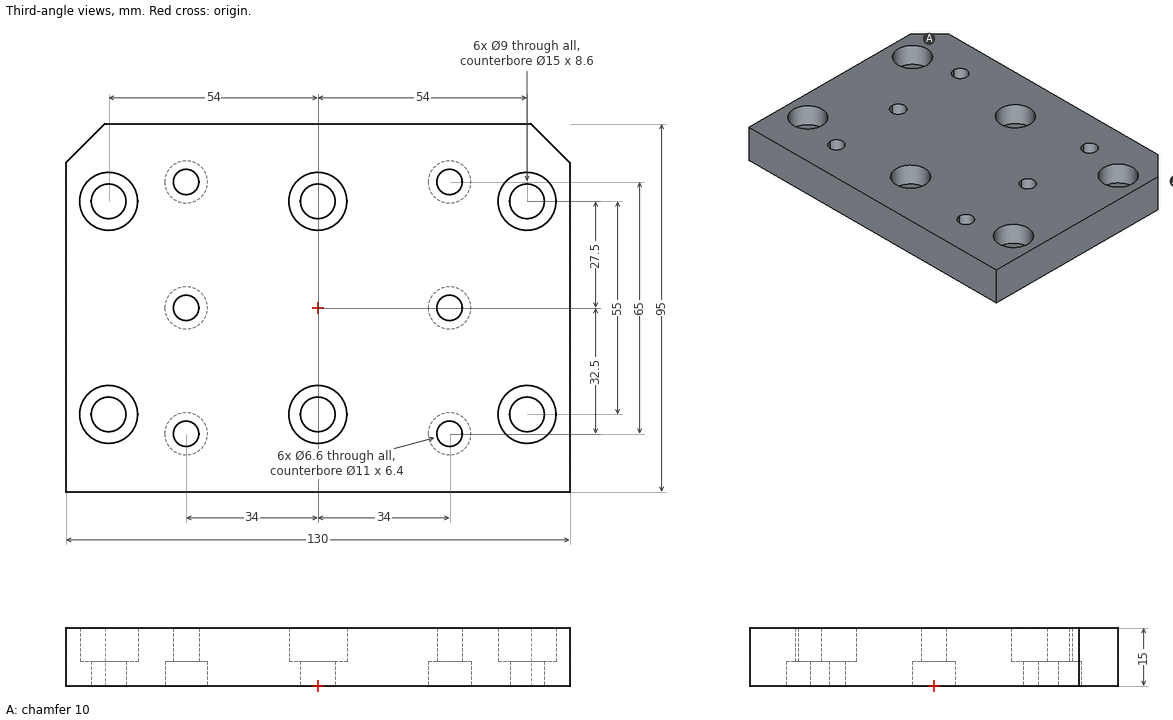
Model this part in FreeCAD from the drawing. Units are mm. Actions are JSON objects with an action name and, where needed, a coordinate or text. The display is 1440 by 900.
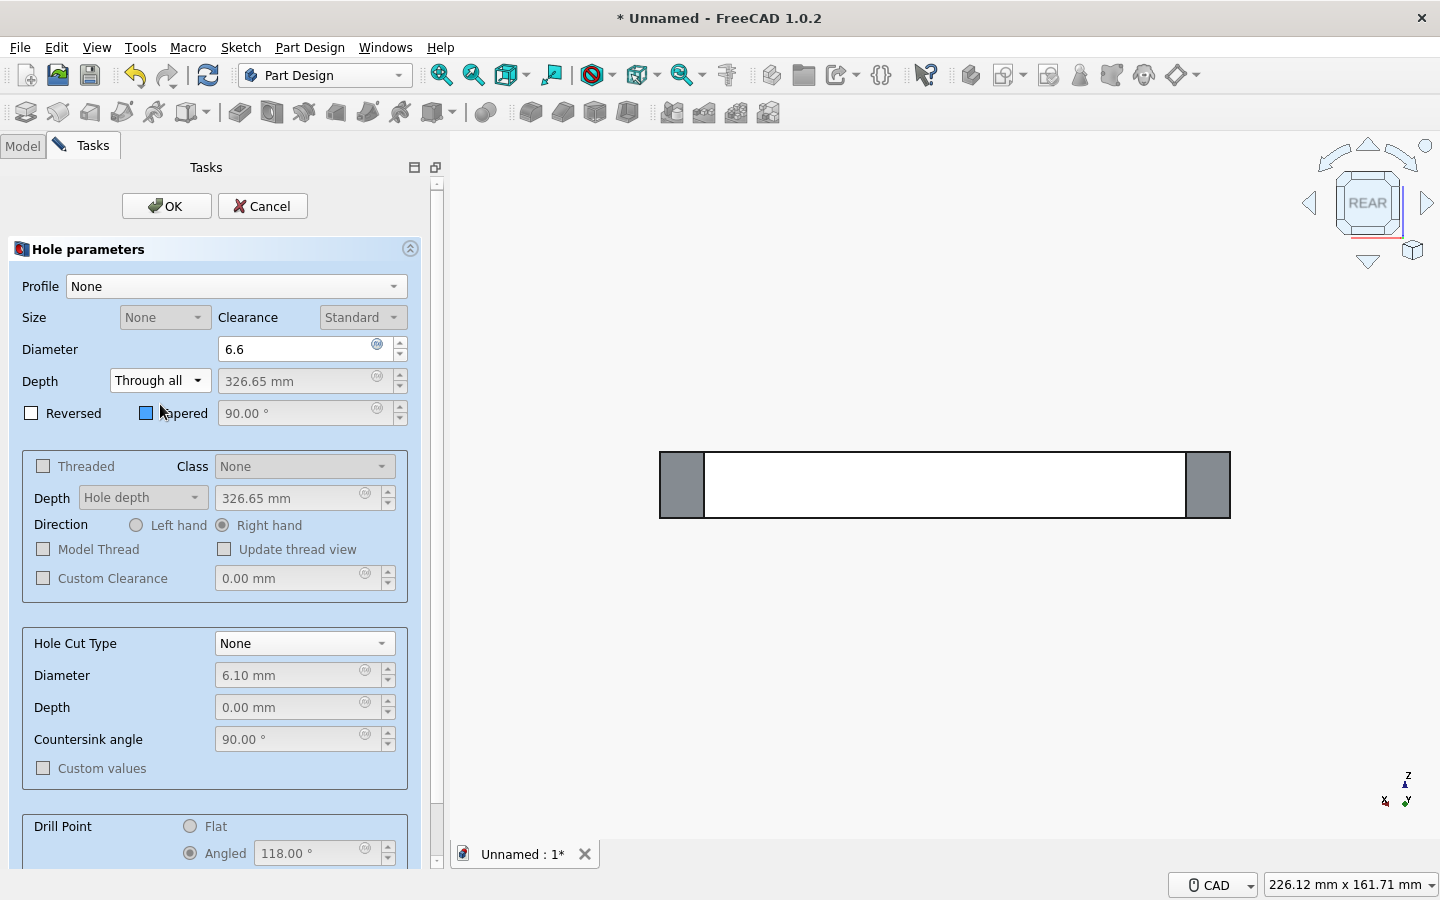
{"action": "left_click", "coordinate": [30, 413]}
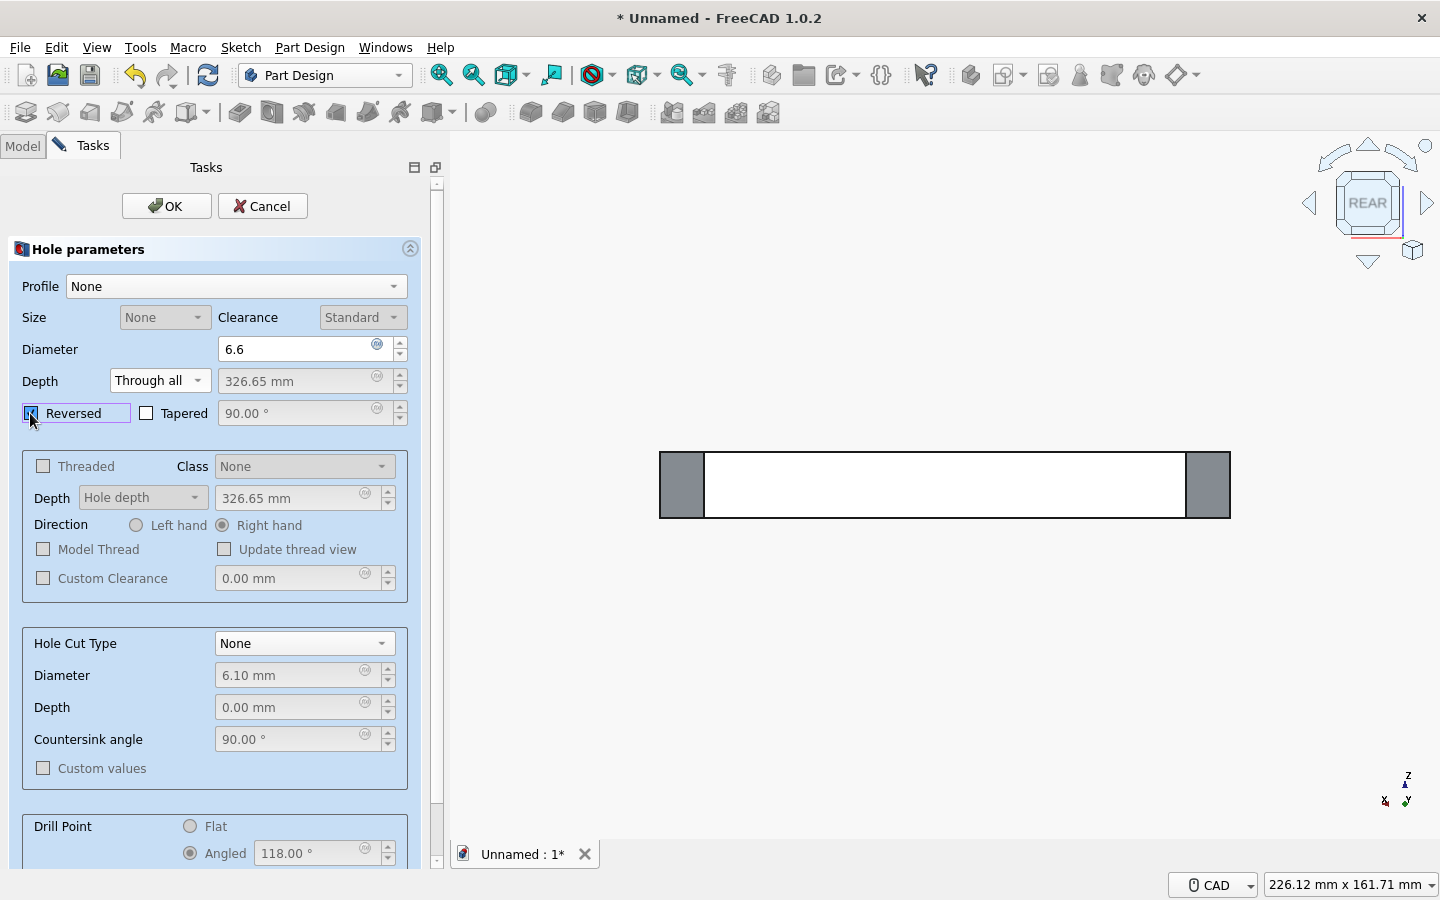
{"action": "left_click", "coordinate": [306, 644]}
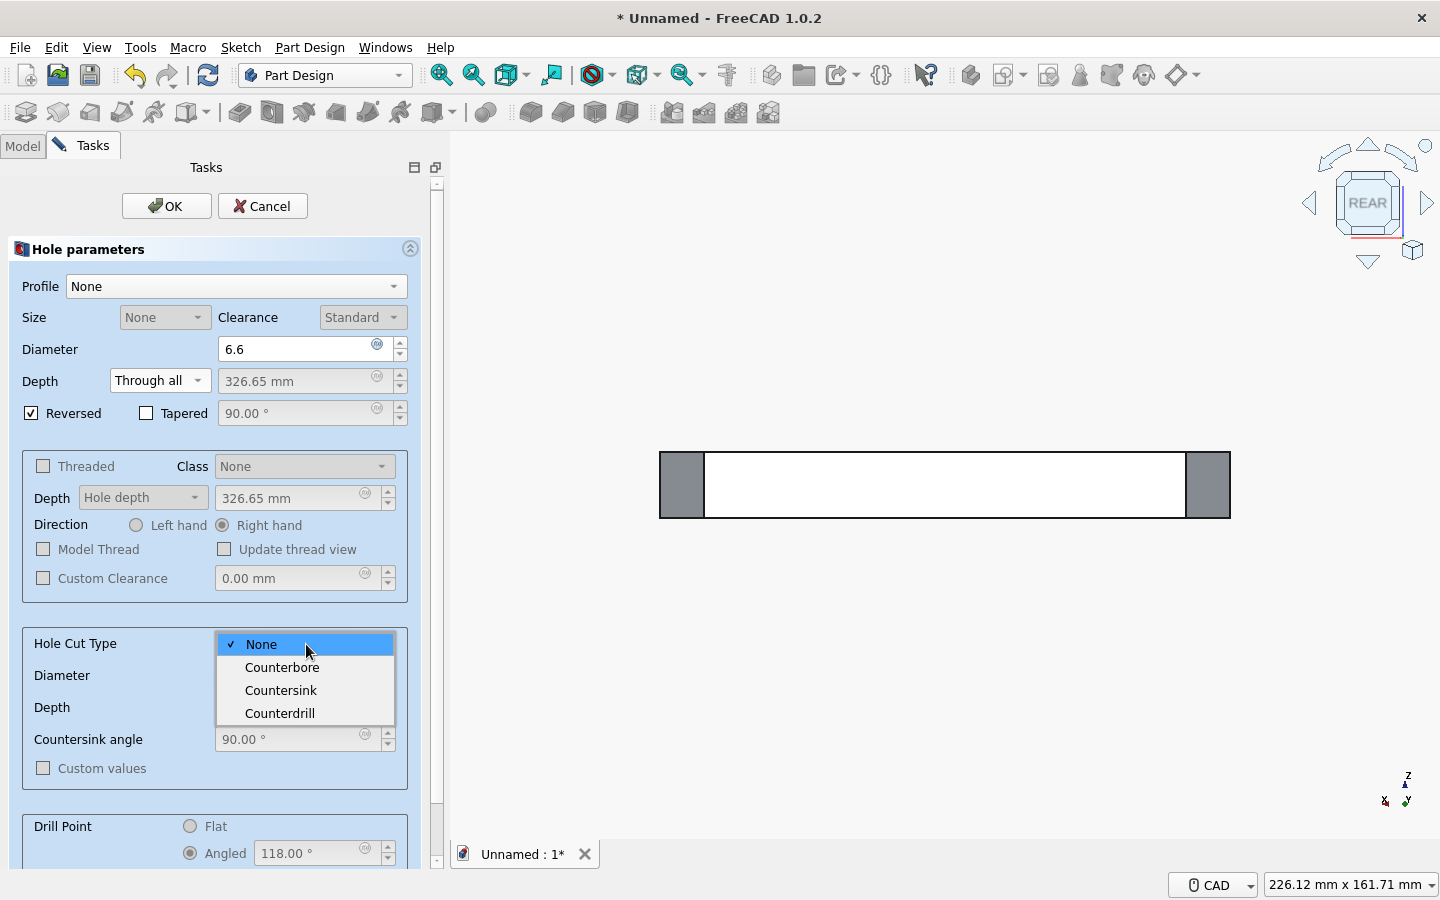
{"action": "left_click", "coordinate": [304, 668]}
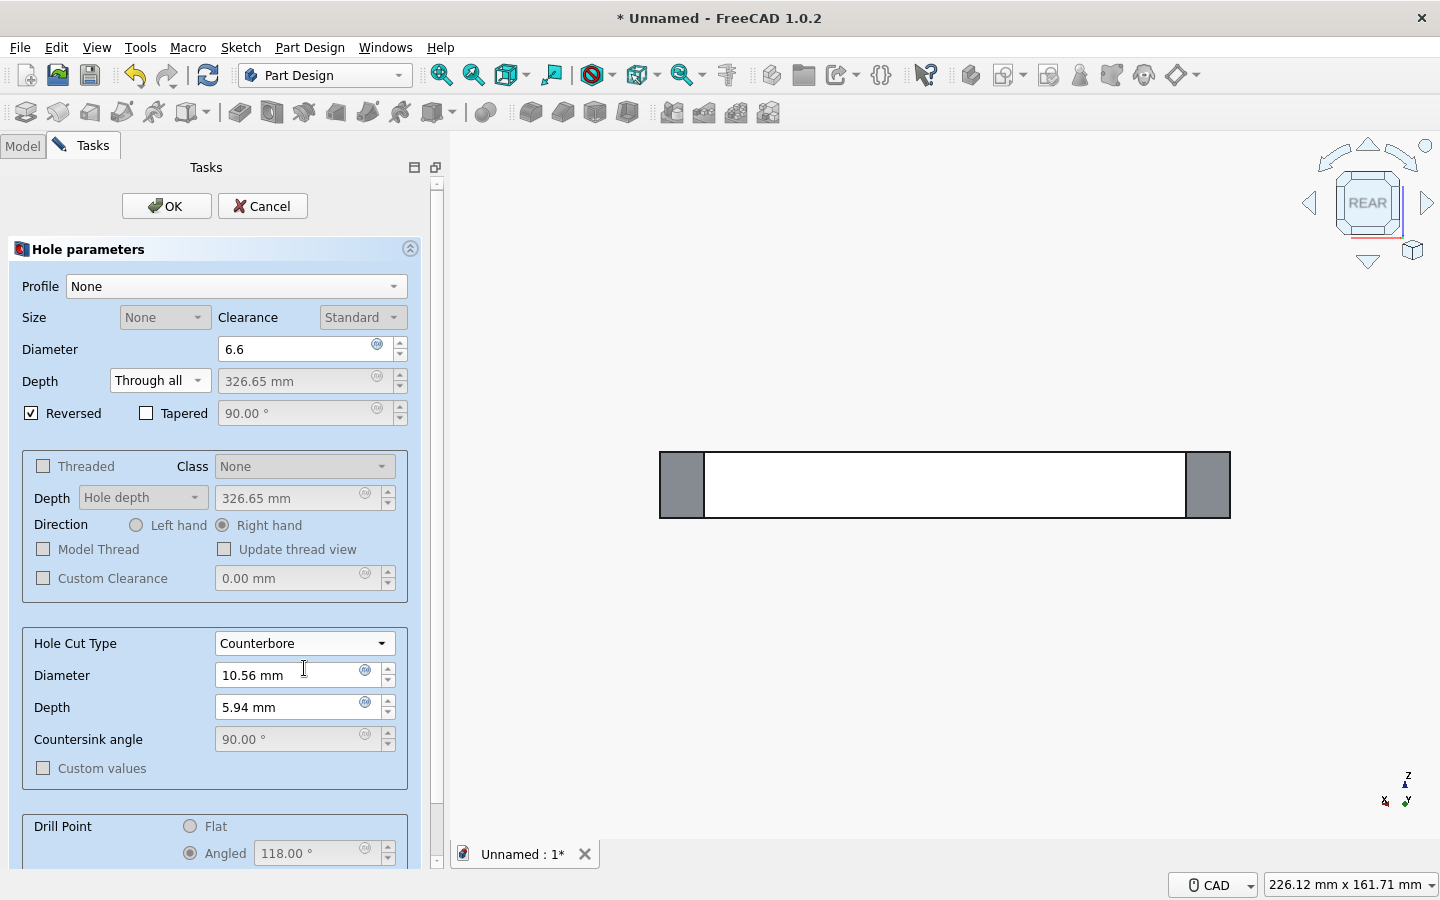
{"action": "triple_click", "coordinate": [298, 675]}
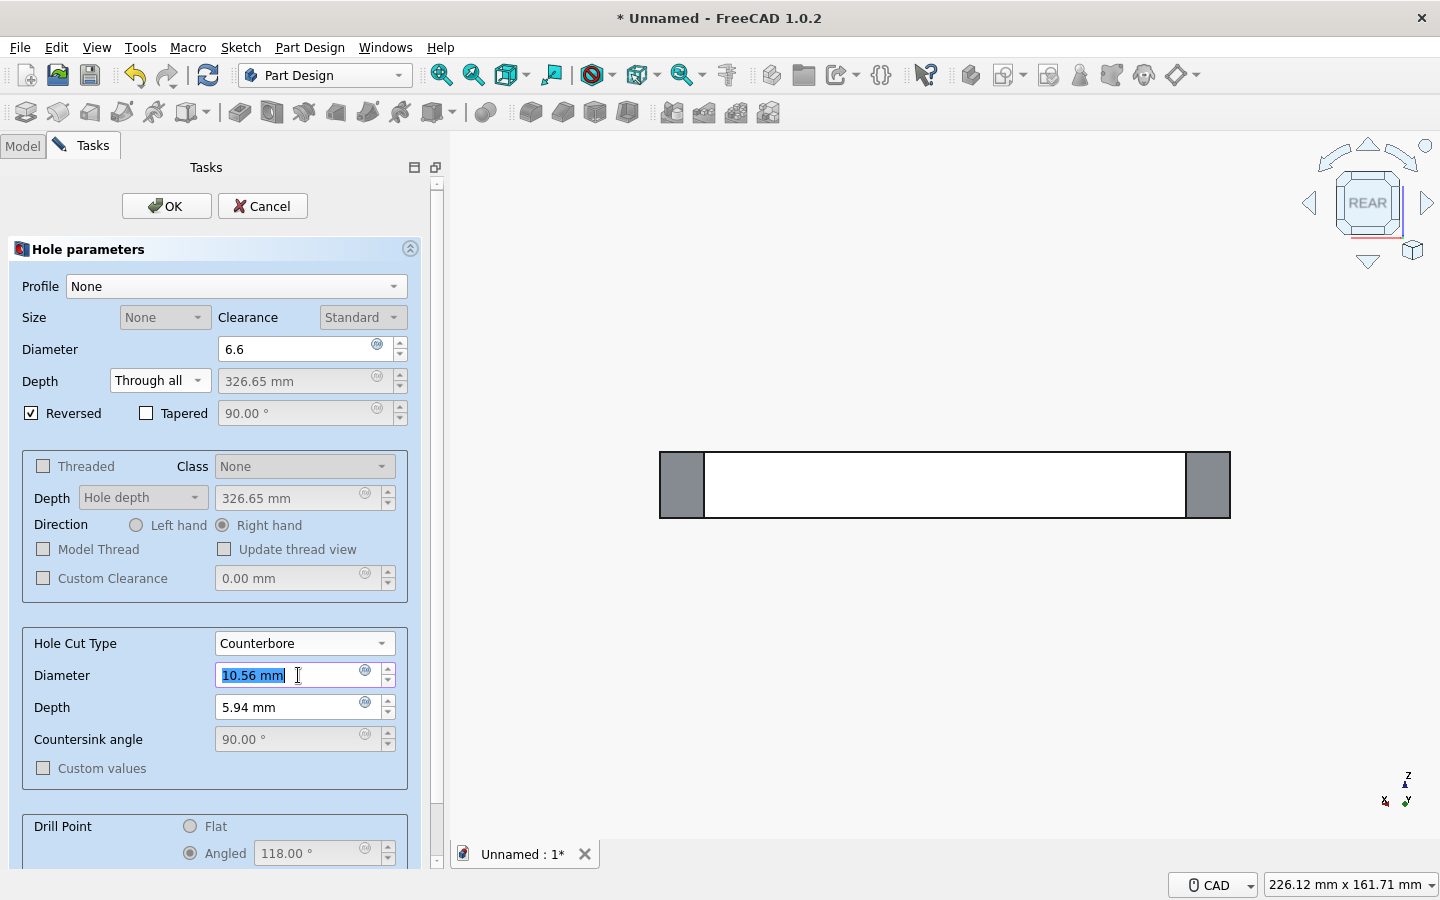
{"action": "type", "text": "11"}
{"action": "key", "text": "Tab"}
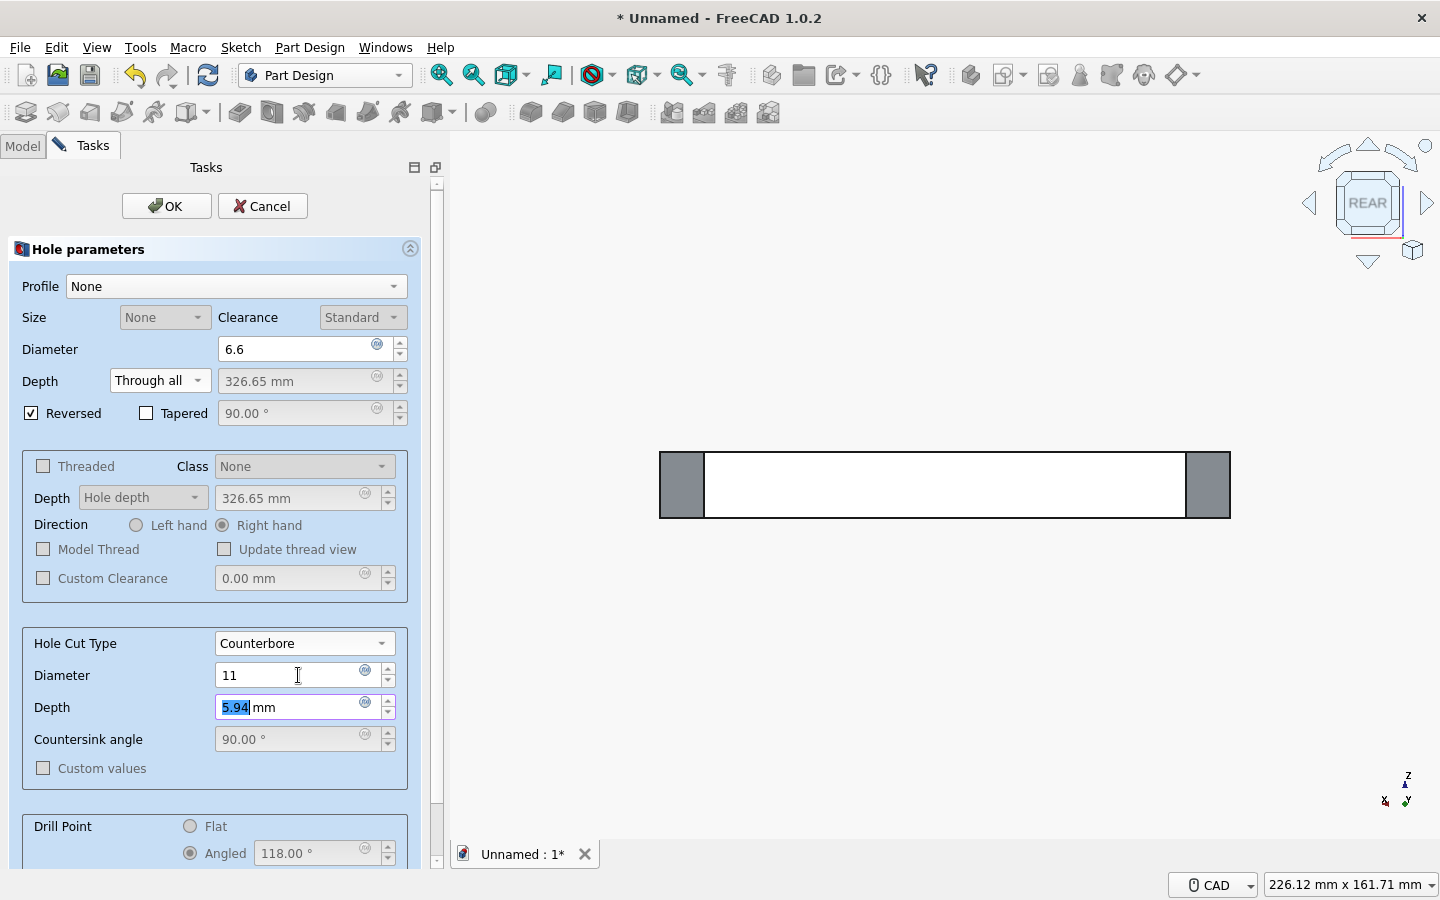
{"action": "type", "text": "6.4"}
{"action": "key", "text": "Tab"}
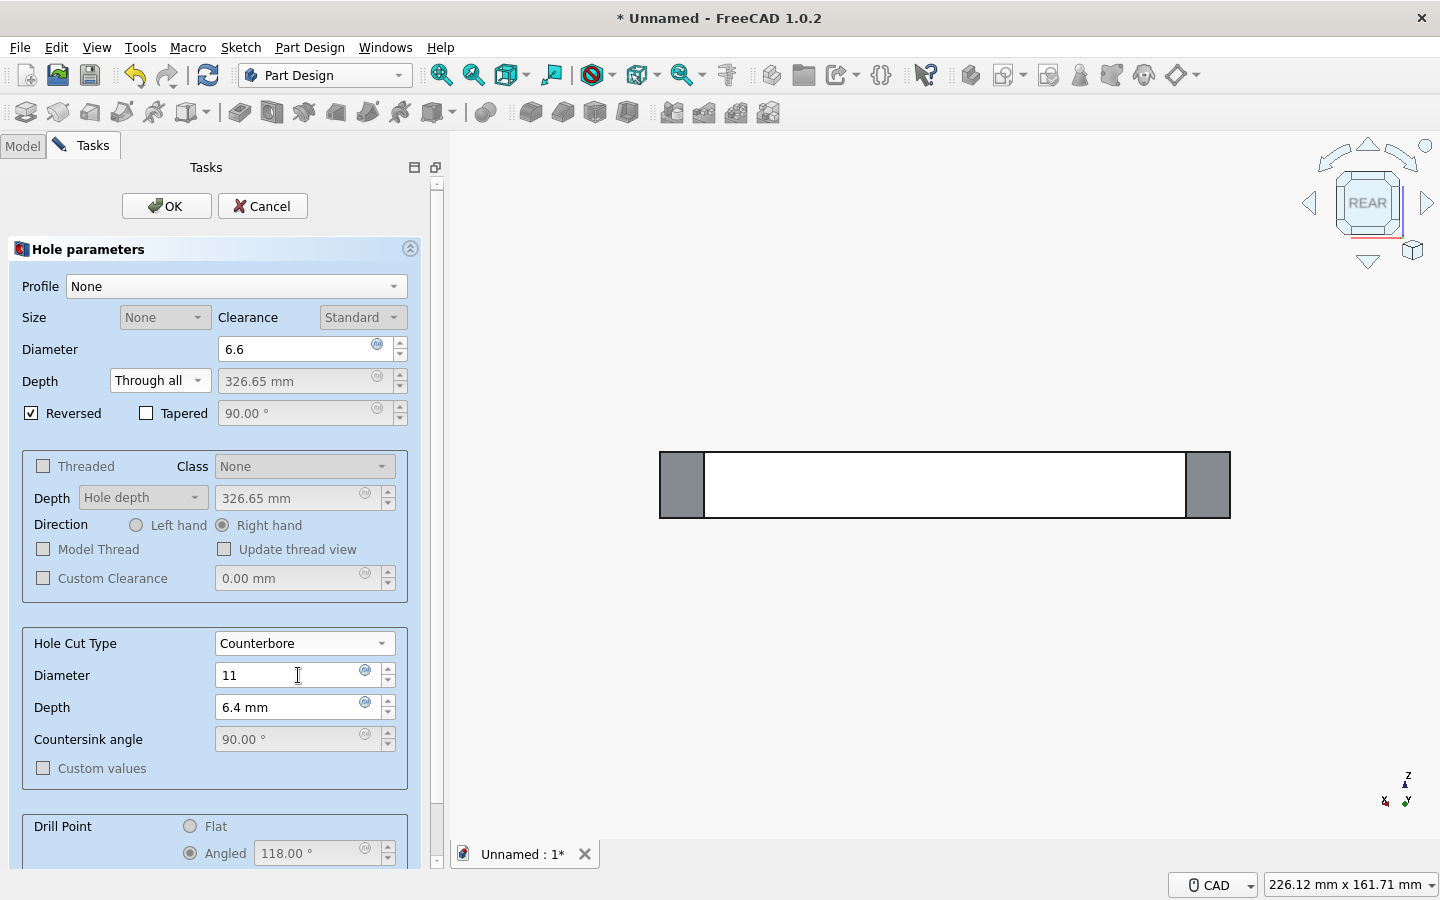
{"action": "left_click", "coordinate": [167, 206]}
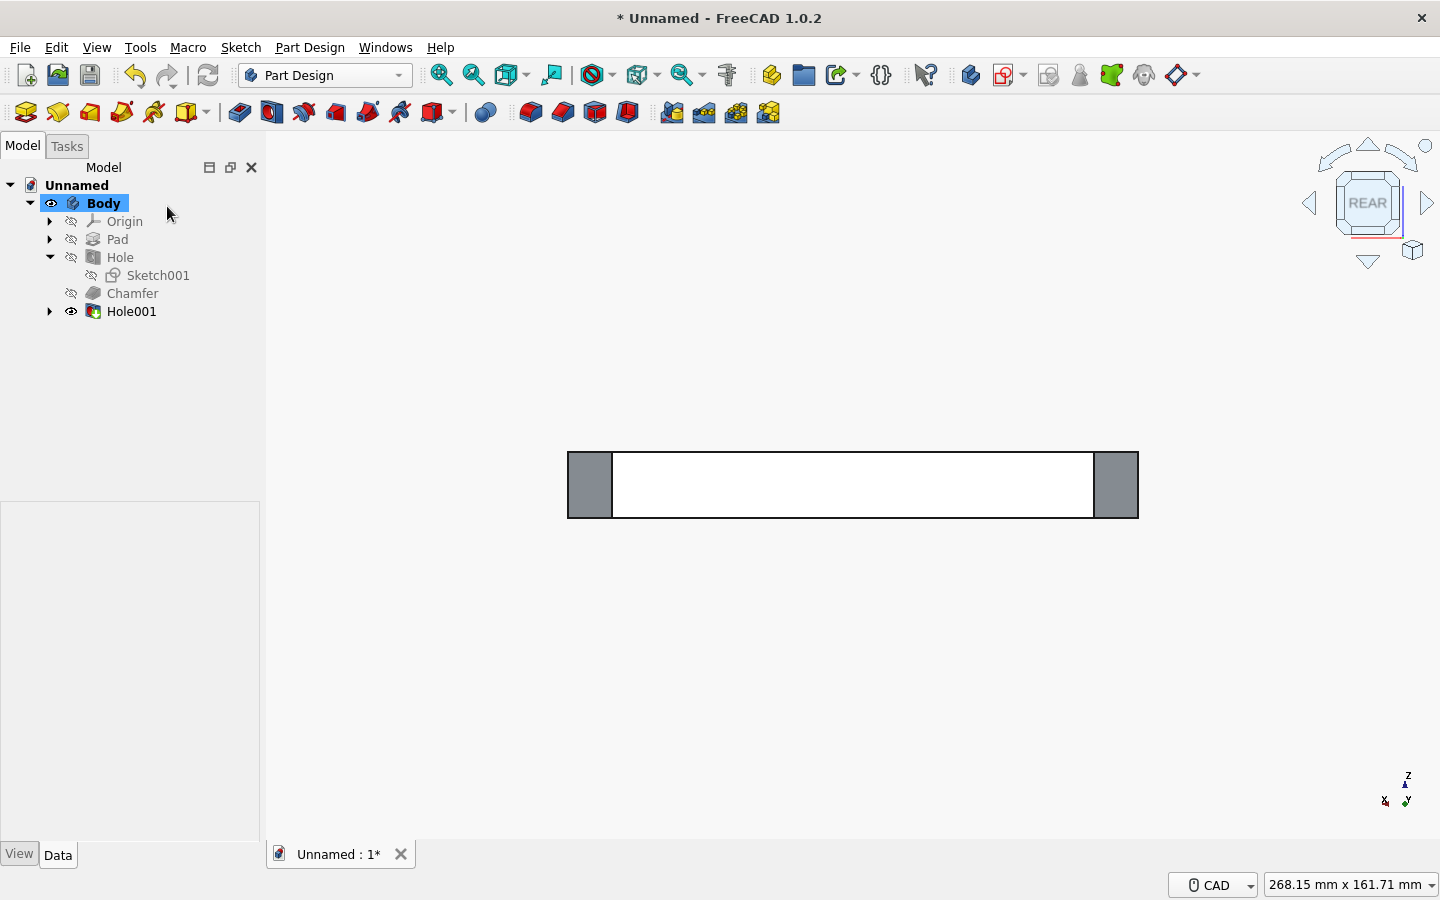
{"action": "key", "text": "0"}